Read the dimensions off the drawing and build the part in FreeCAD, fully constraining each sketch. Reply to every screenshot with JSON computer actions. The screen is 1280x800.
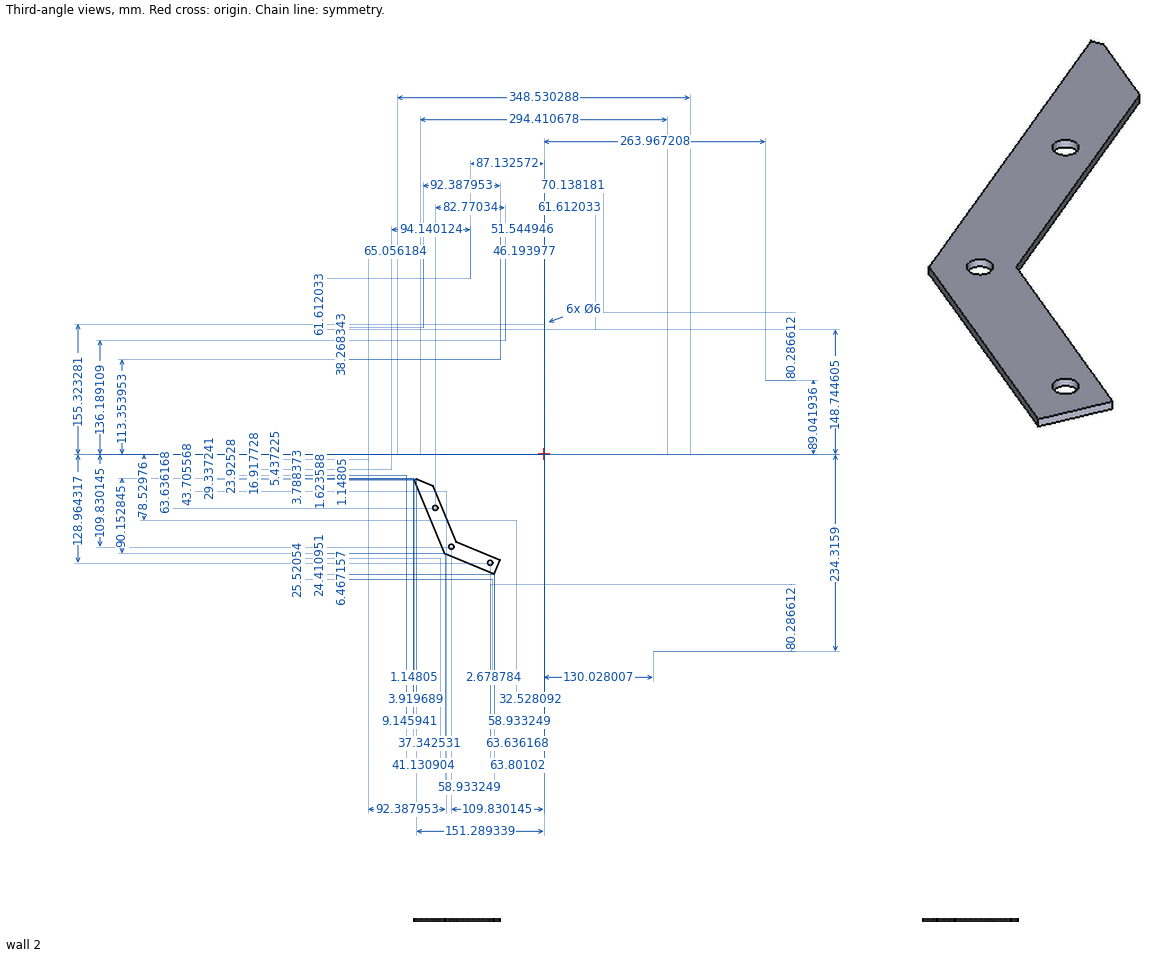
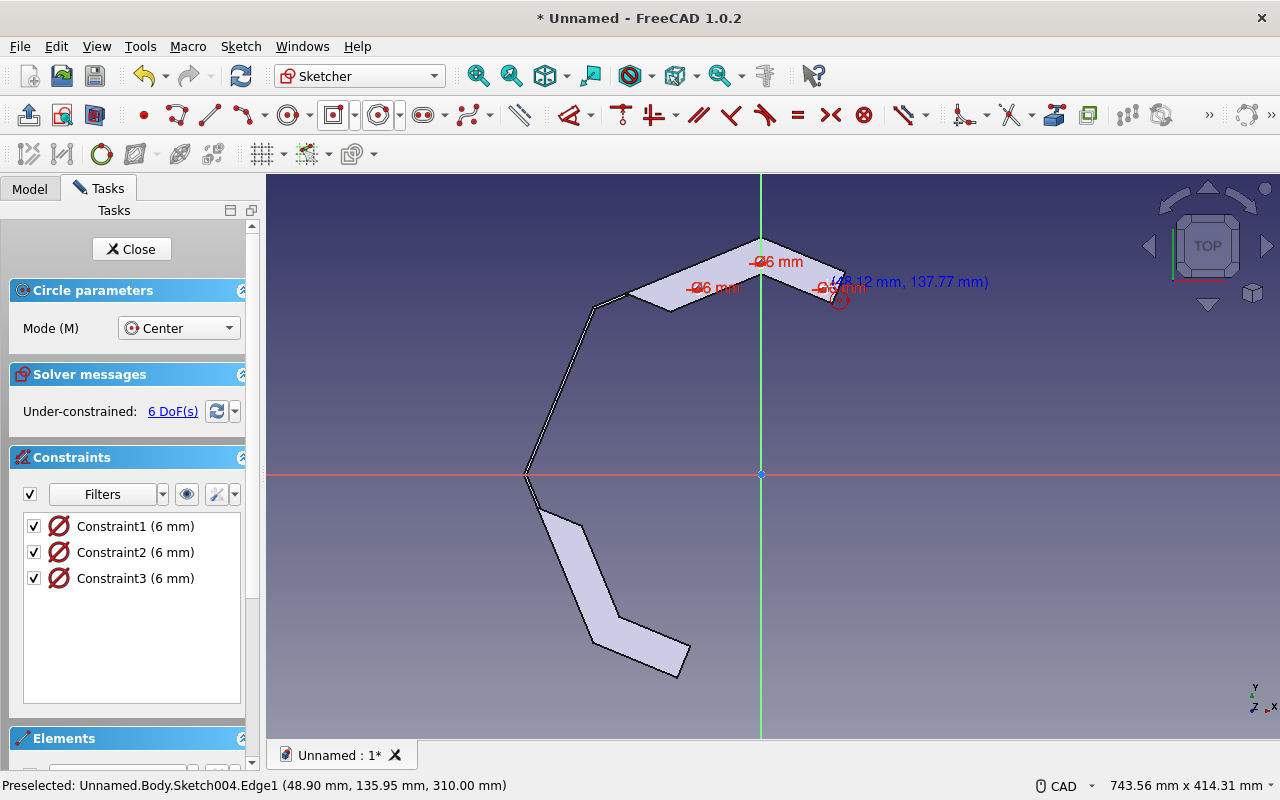
{"action": "scroll", "coordinate": [586, 562], "scroll_direction": "up", "scroll_amount": 9}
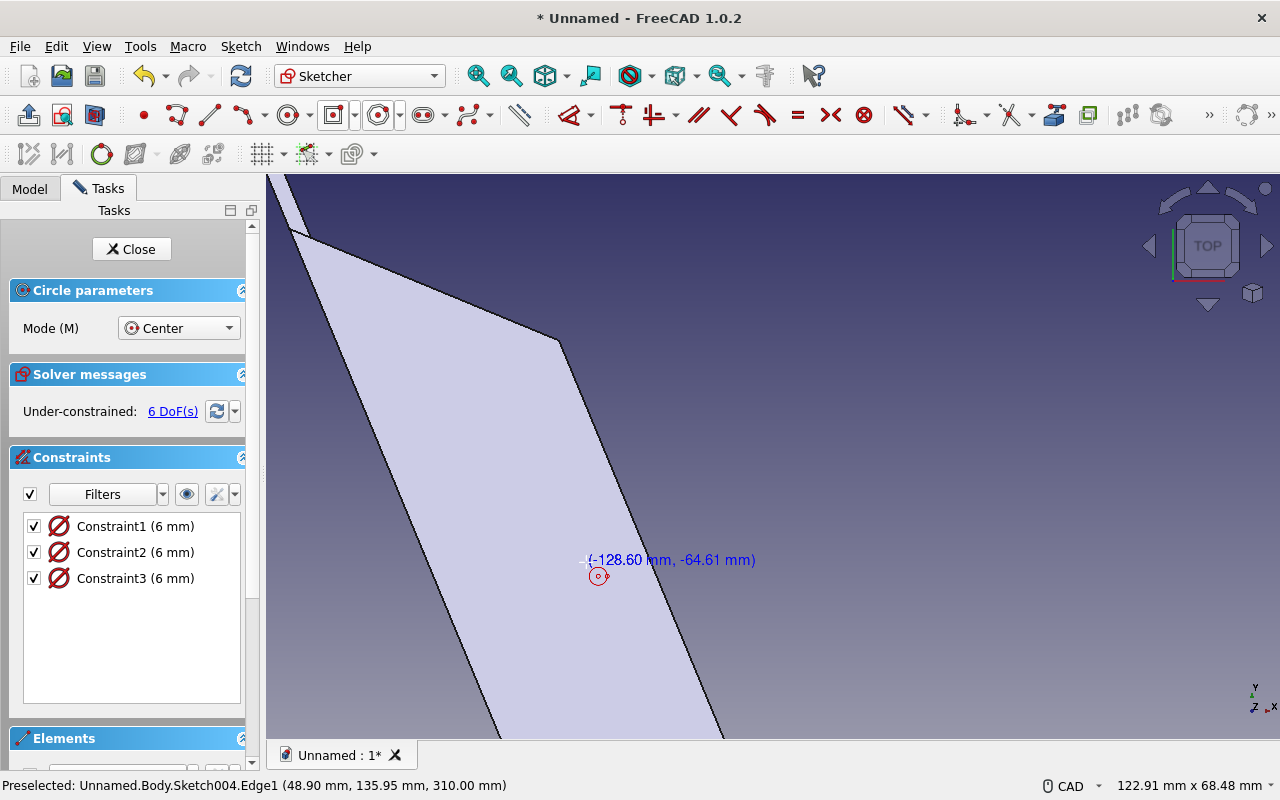
{"action": "scroll", "coordinate": [586, 562], "scroll_direction": "down", "scroll_amount": 9}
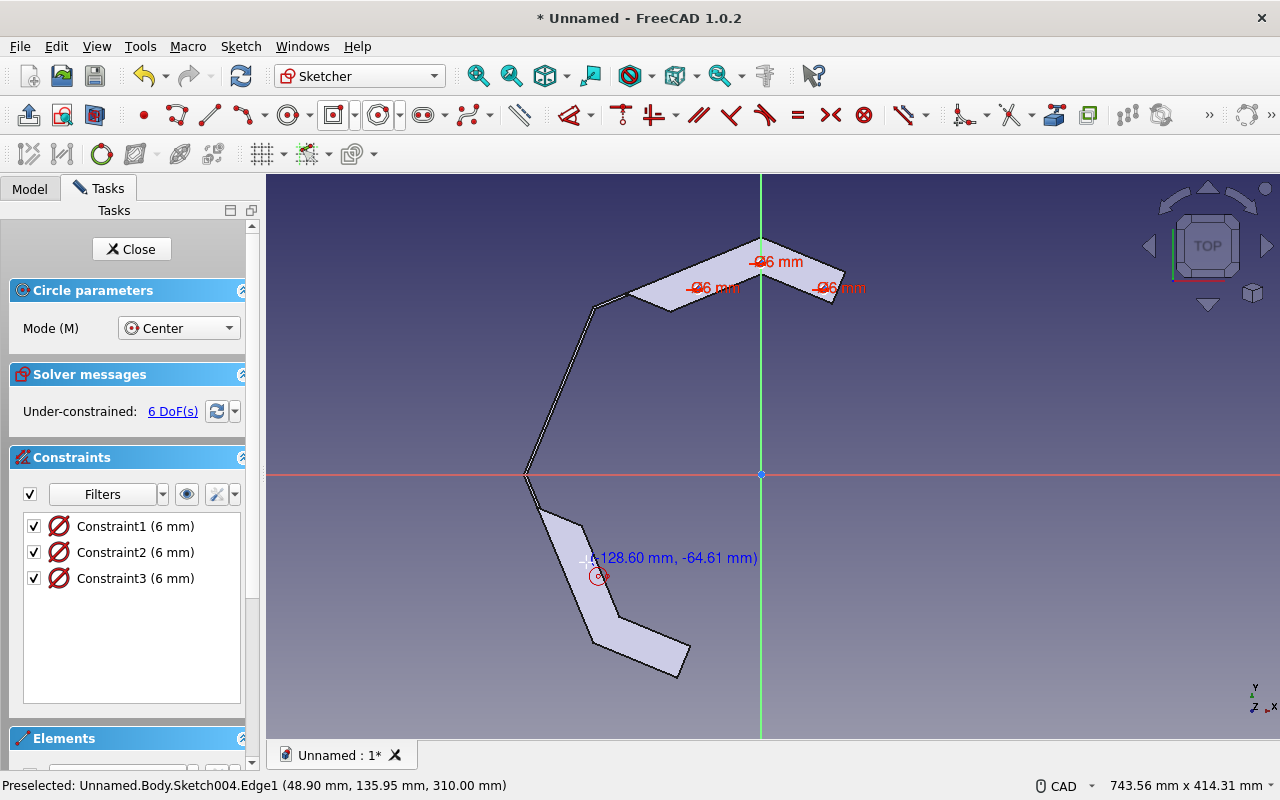
{"action": "left_click", "coordinate": [586, 562]}
{"action": "mouse_move", "coordinate": [588, 559]}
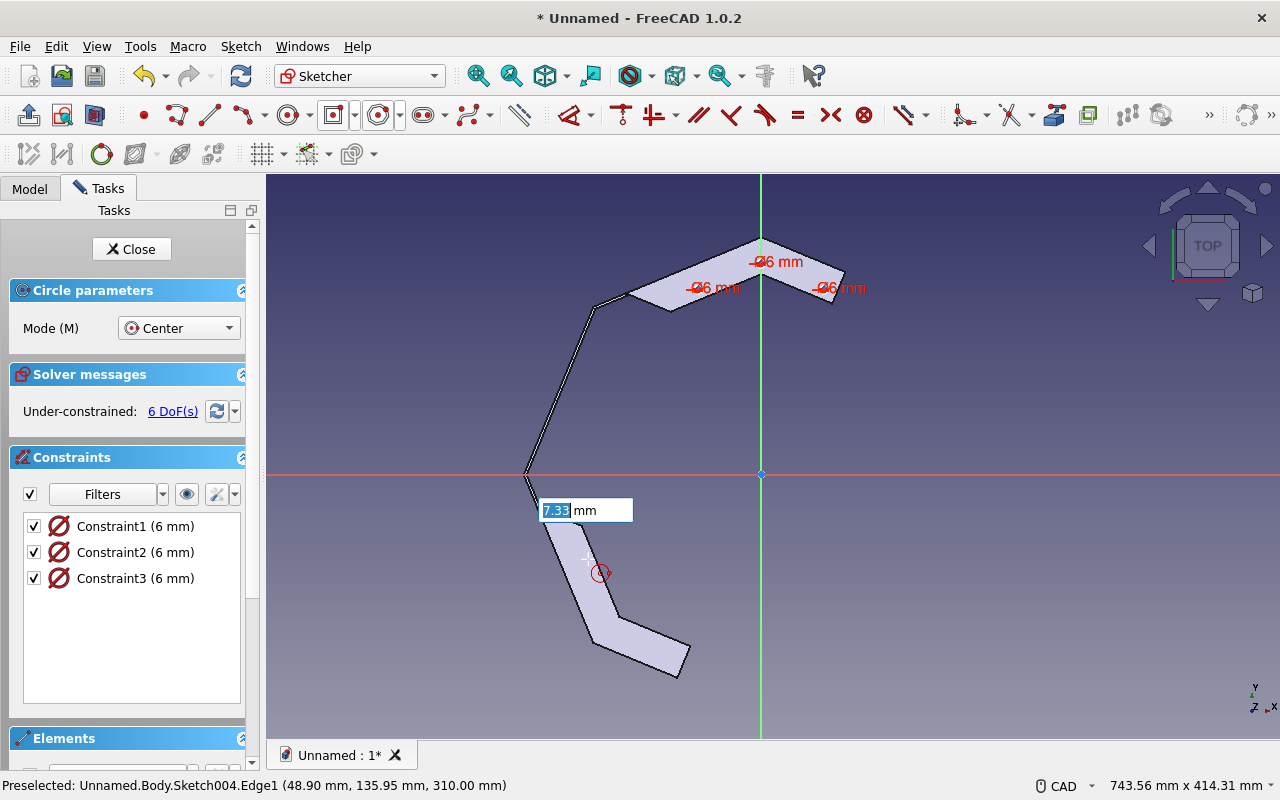
{"action": "type", "text": "6"}
{"action": "key", "text": "Return"}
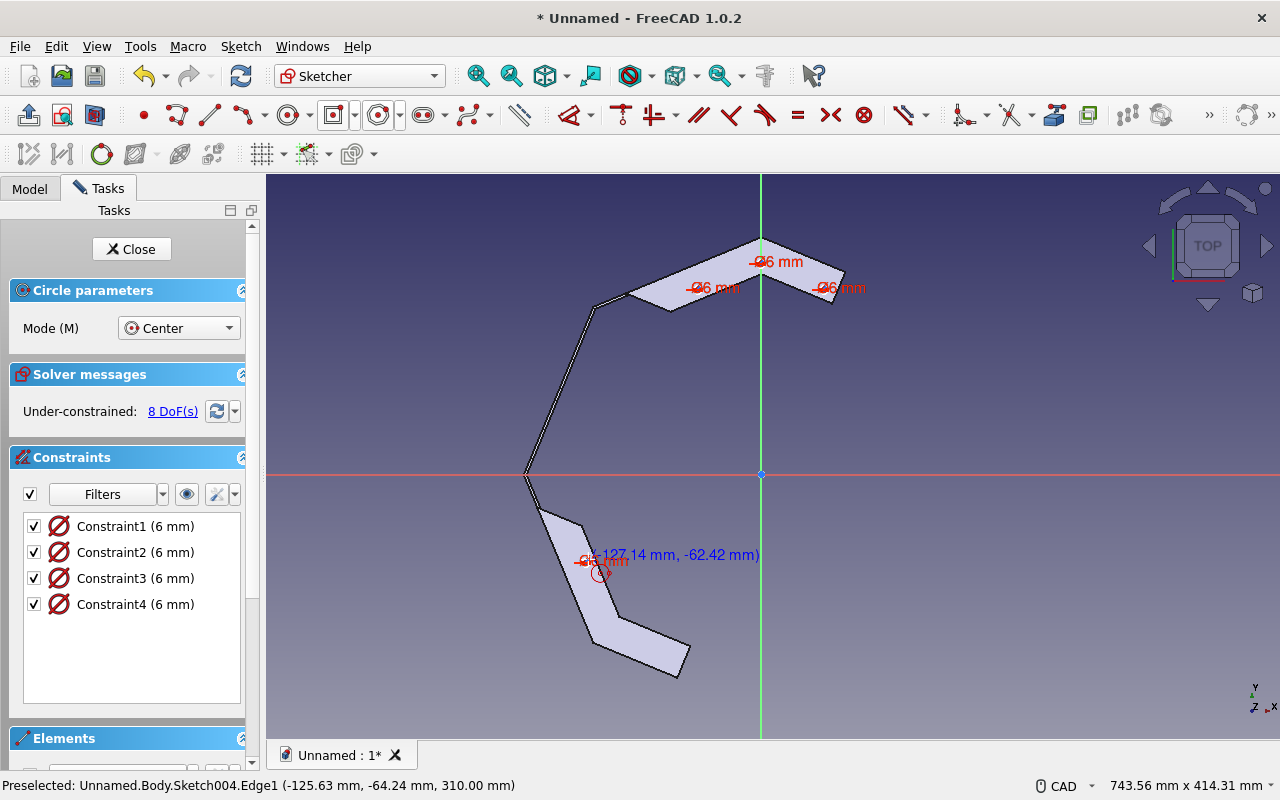
{"action": "scroll", "coordinate": [612, 625], "scroll_direction": "up", "scroll_amount": 9}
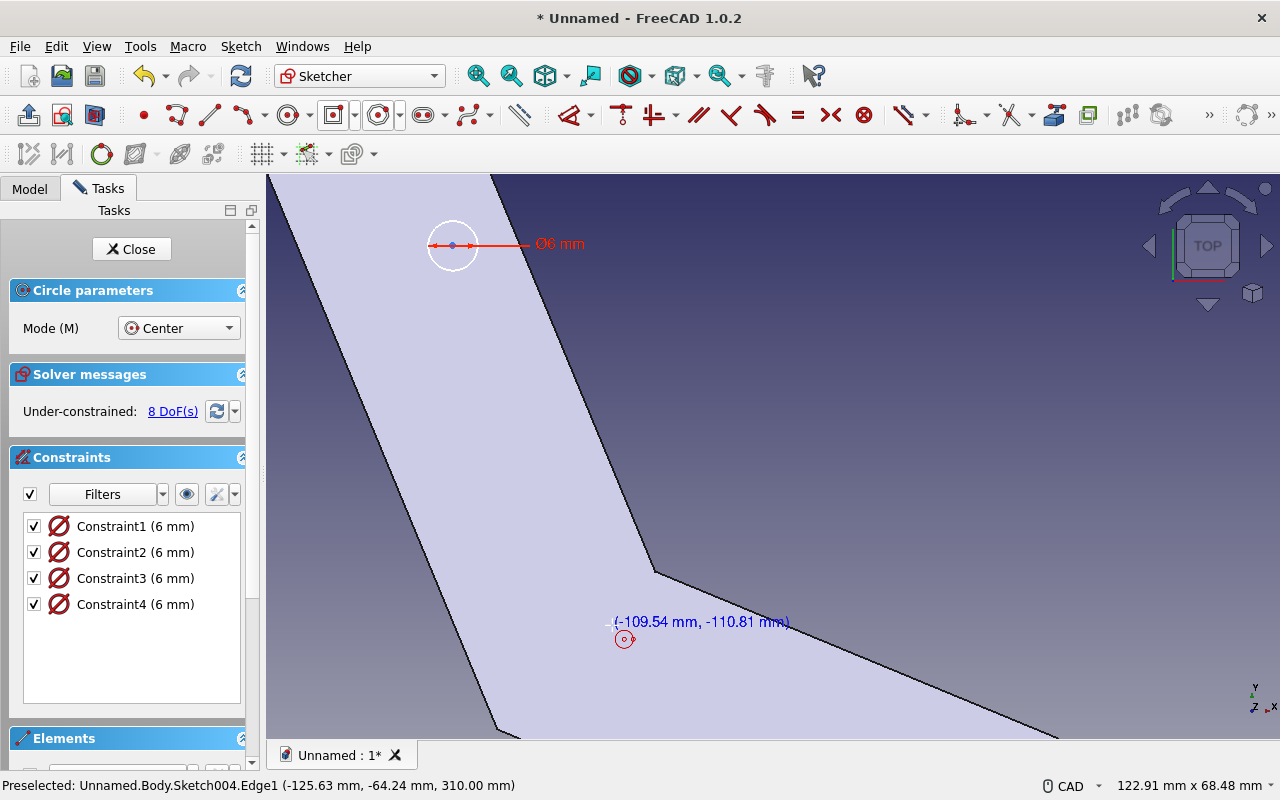
{"action": "scroll", "coordinate": [612, 625], "scroll_direction": "down", "scroll_amount": 9}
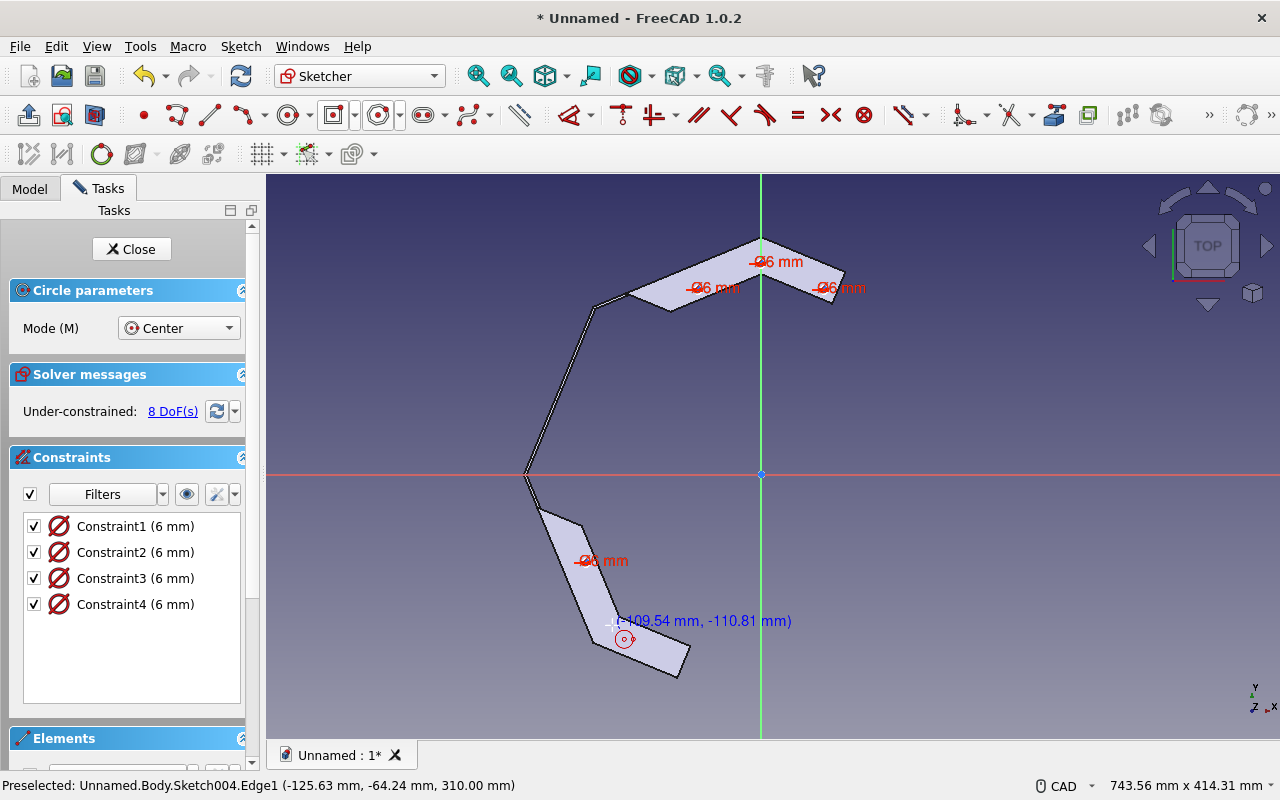
{"action": "left_click", "coordinate": [612, 625]}
{"action": "mouse_move", "coordinate": [614, 622]}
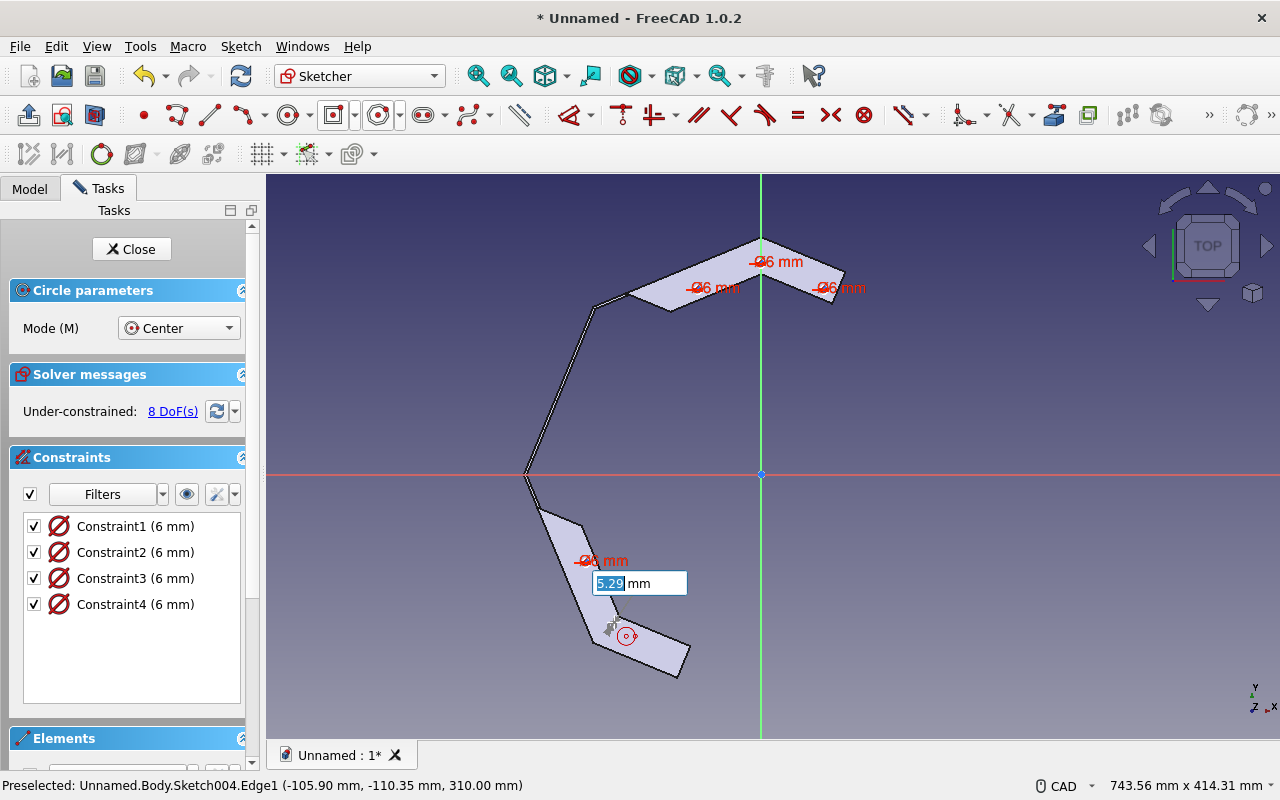
{"action": "type", "text": "6"}
{"action": "key", "text": "Return"}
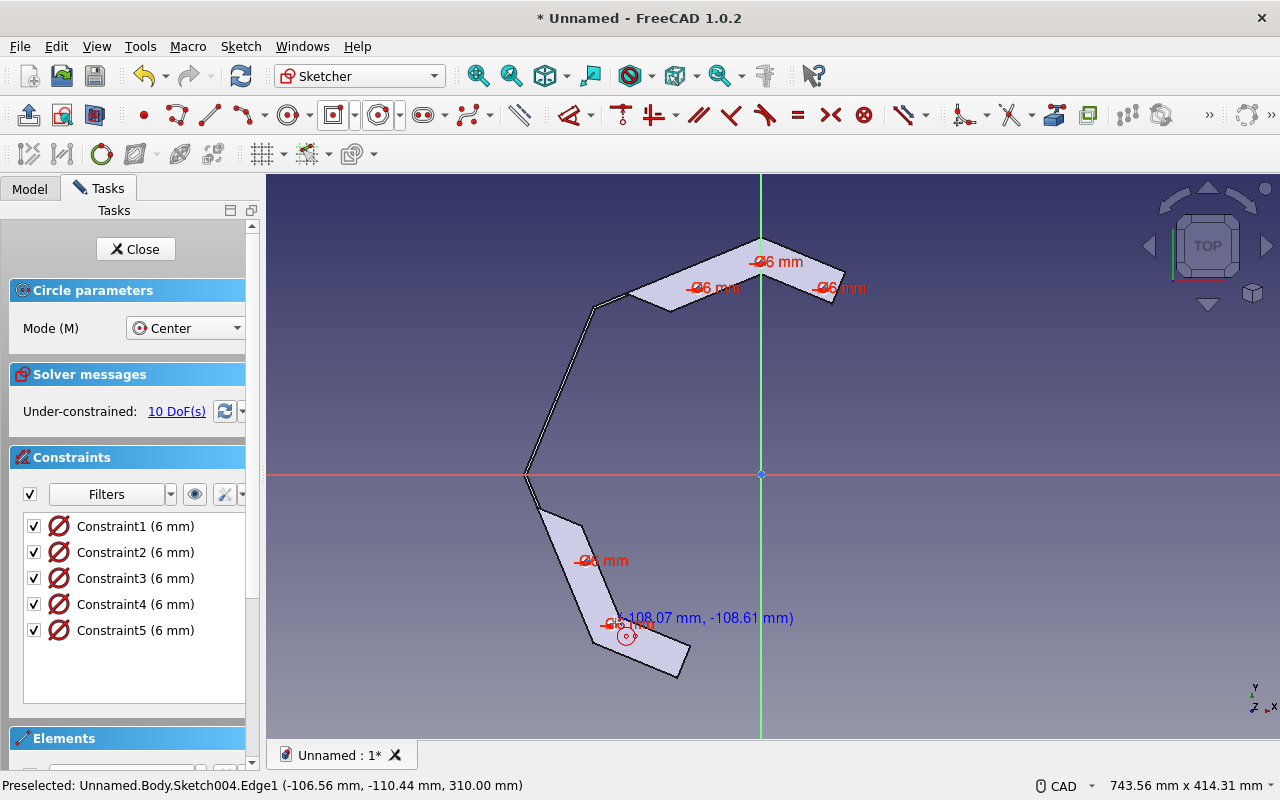
{"action": "scroll", "coordinate": [675, 651], "scroll_direction": "up", "scroll_amount": 9}